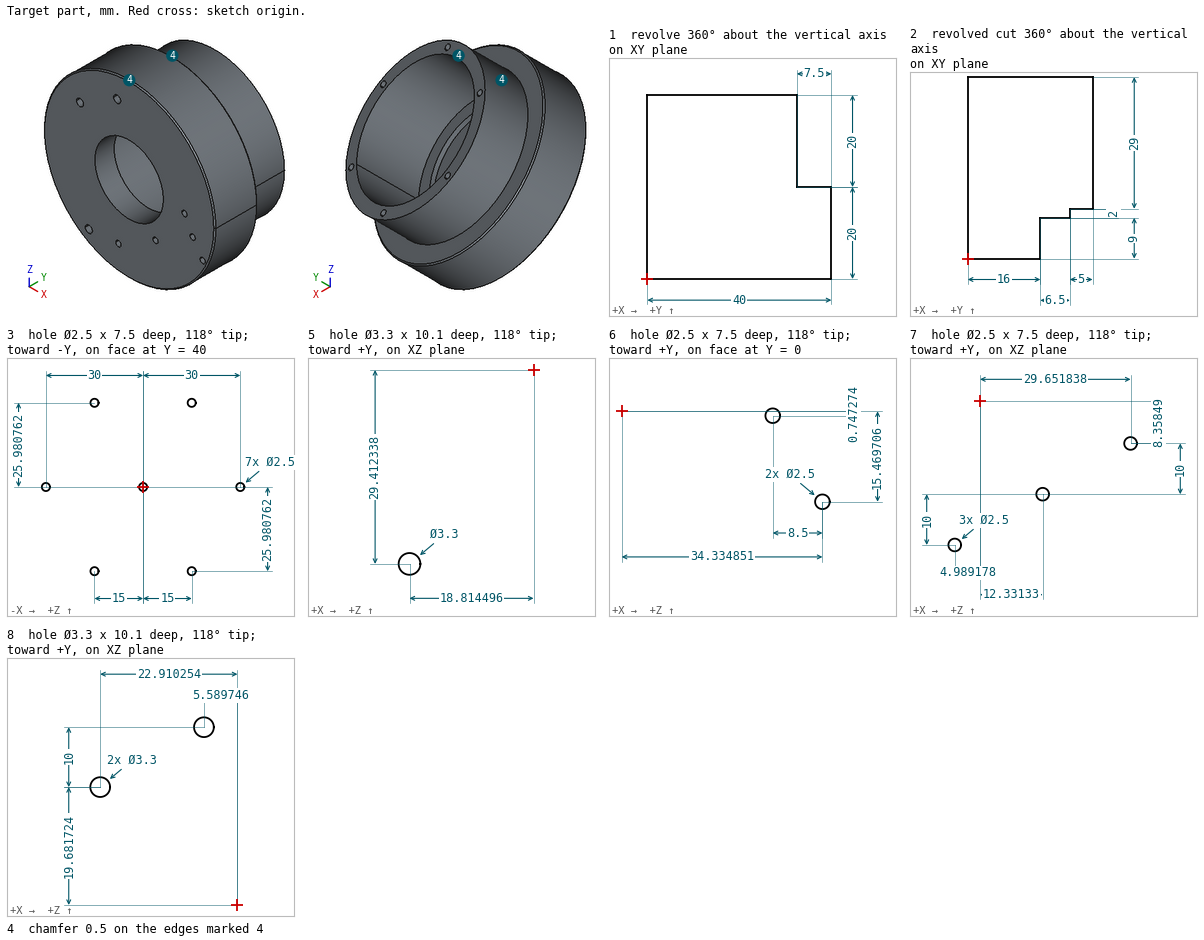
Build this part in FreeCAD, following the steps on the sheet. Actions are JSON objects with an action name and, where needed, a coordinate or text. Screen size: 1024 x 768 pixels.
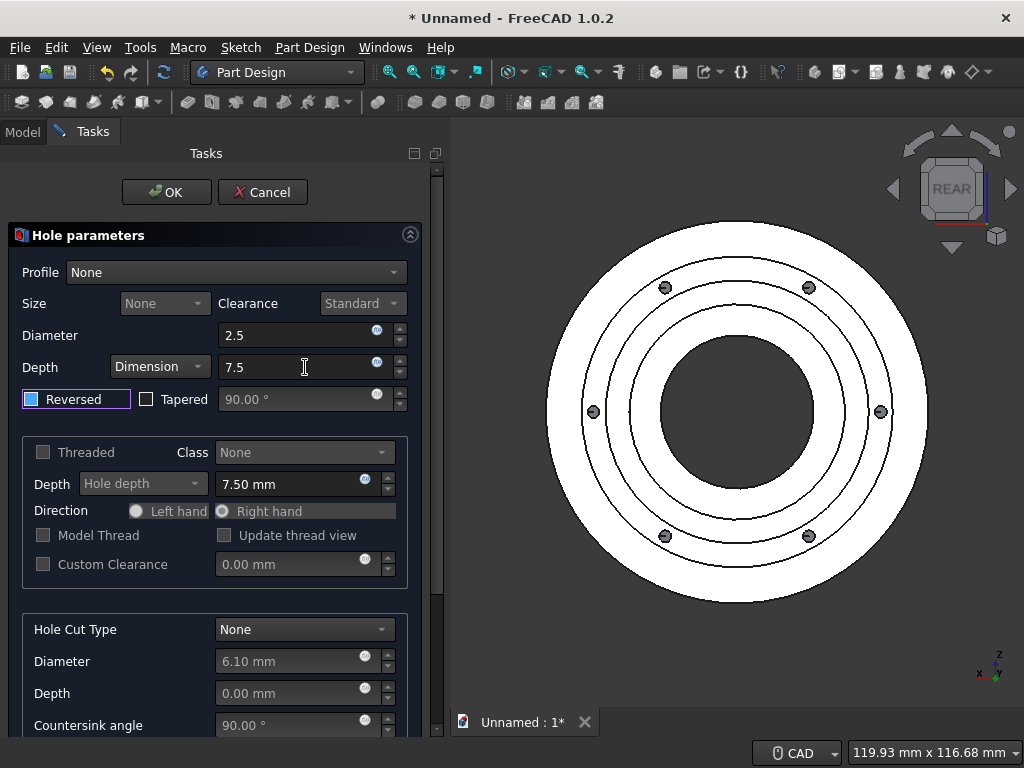
{"action": "left_click", "coordinate": [167, 192]}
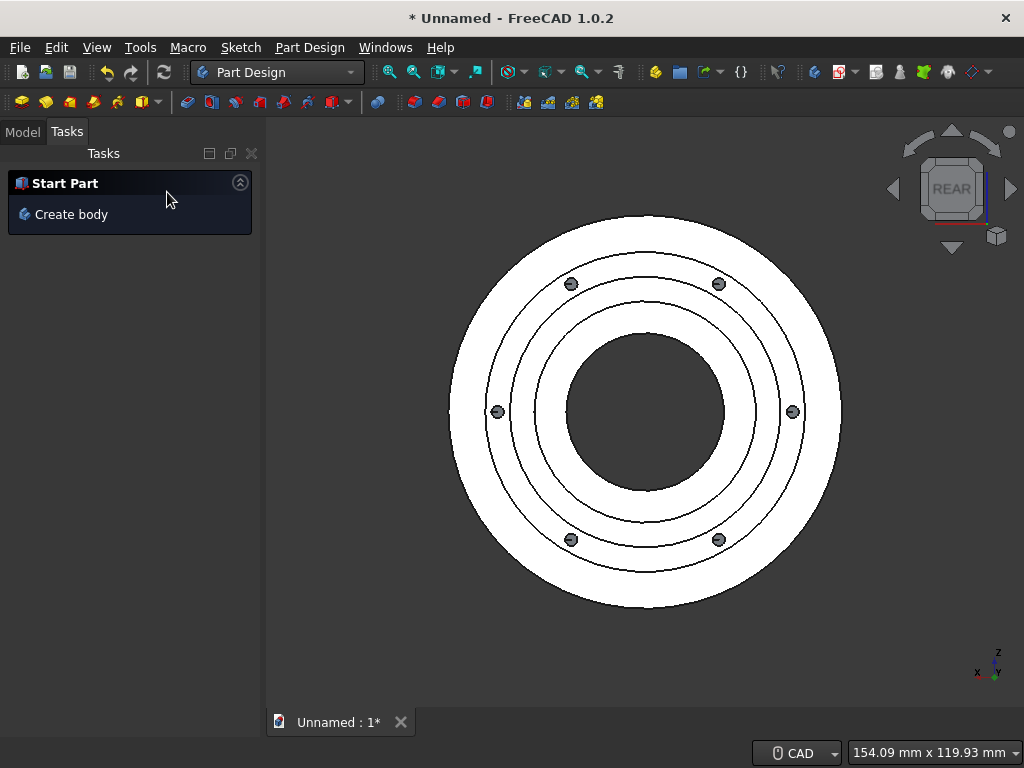
{"action": "left_click", "coordinate": [842, 411]}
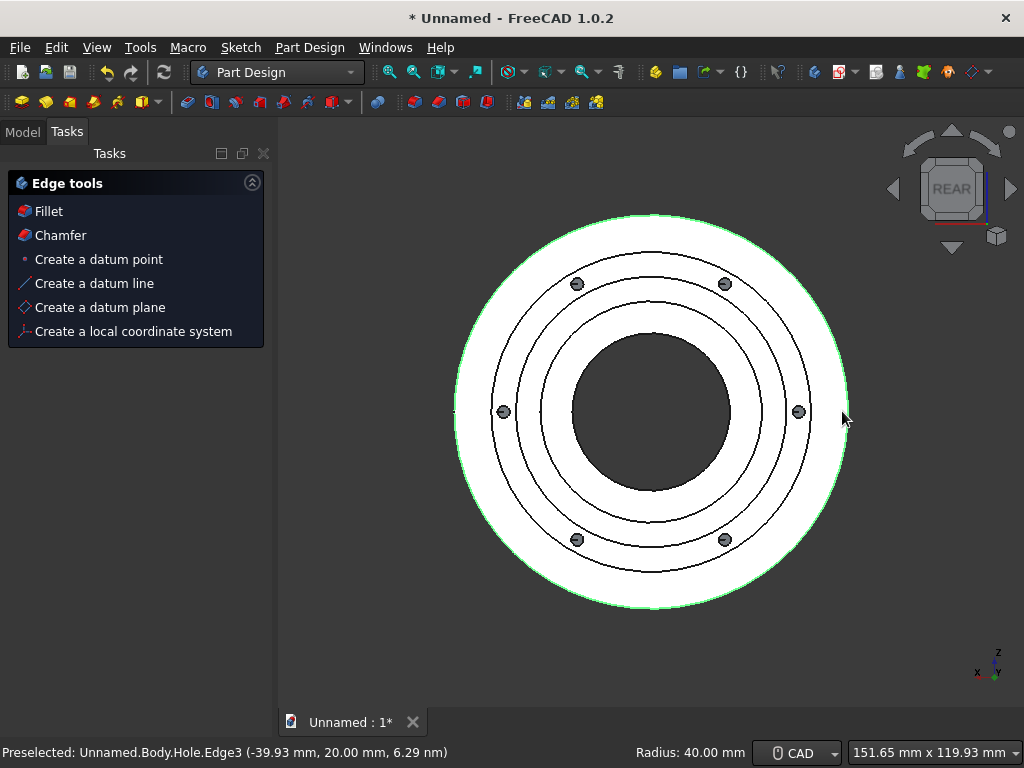
{"action": "key", "text": "0"}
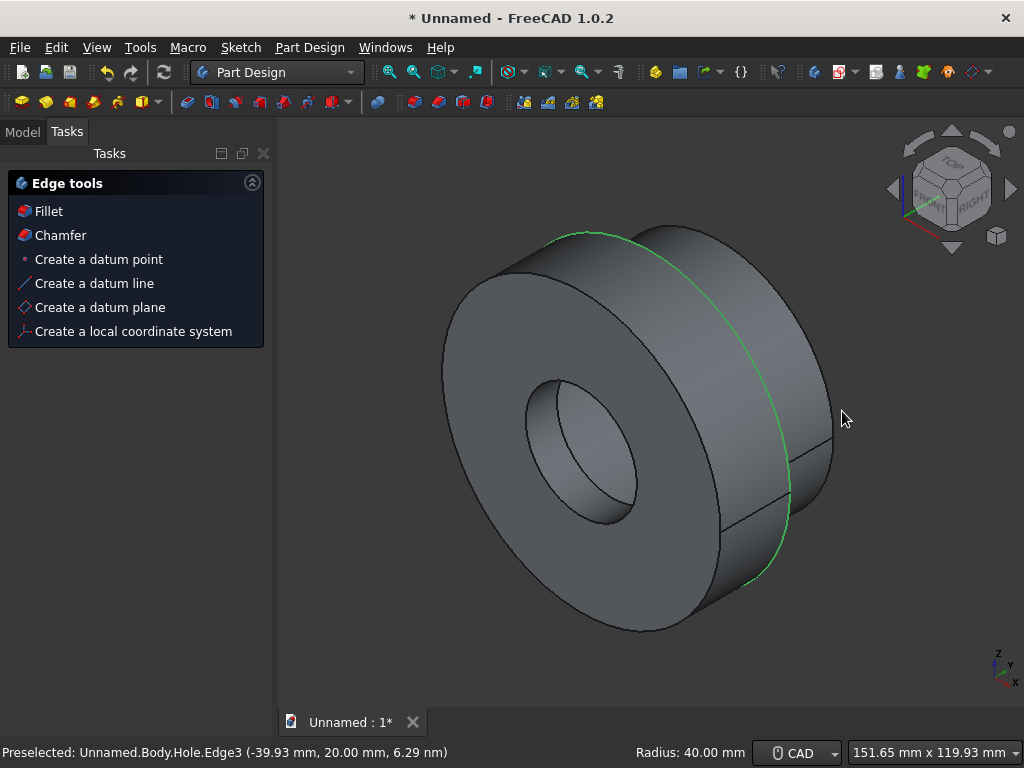
{"action": "left_click", "coordinate": [538, 273], "text": "ctrl"}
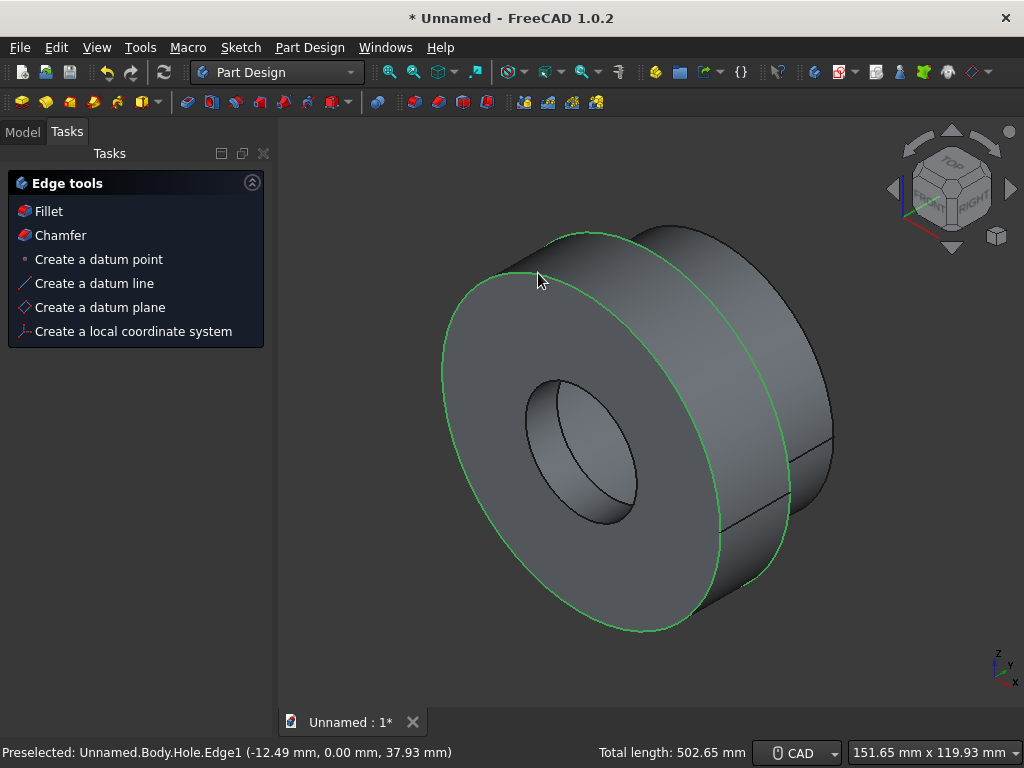
{"action": "left_click", "coordinate": [440, 102]}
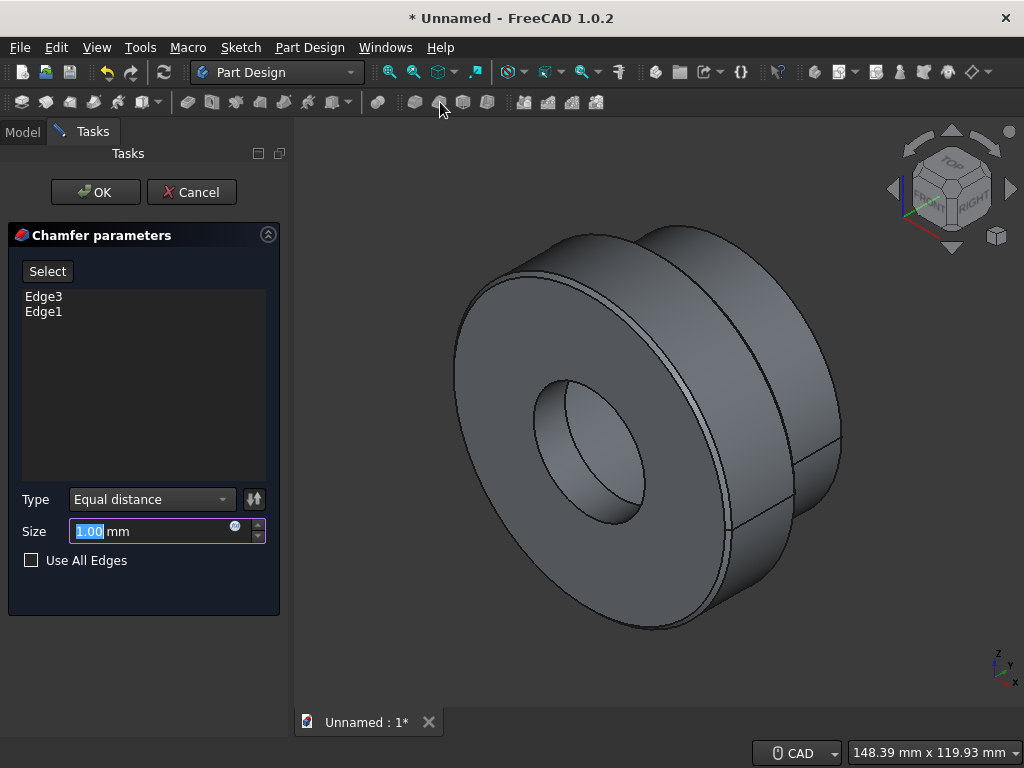
{"action": "type", "text": "0.5"}
{"action": "key", "text": "Tab"}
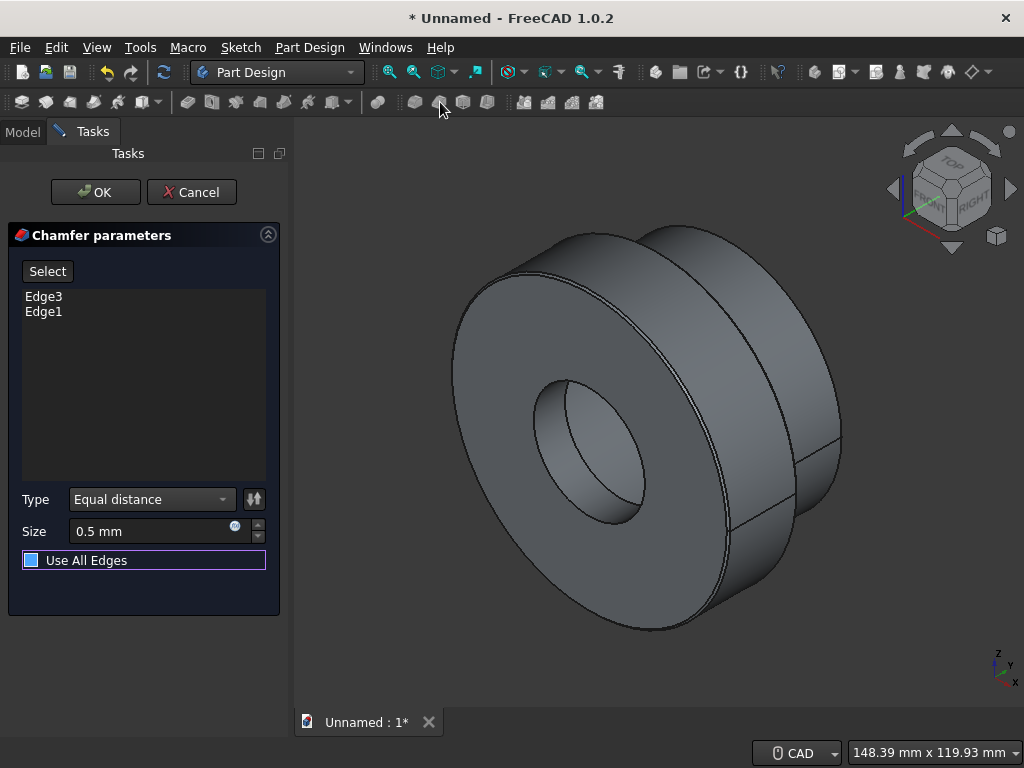
{"action": "left_click", "coordinate": [96, 192]}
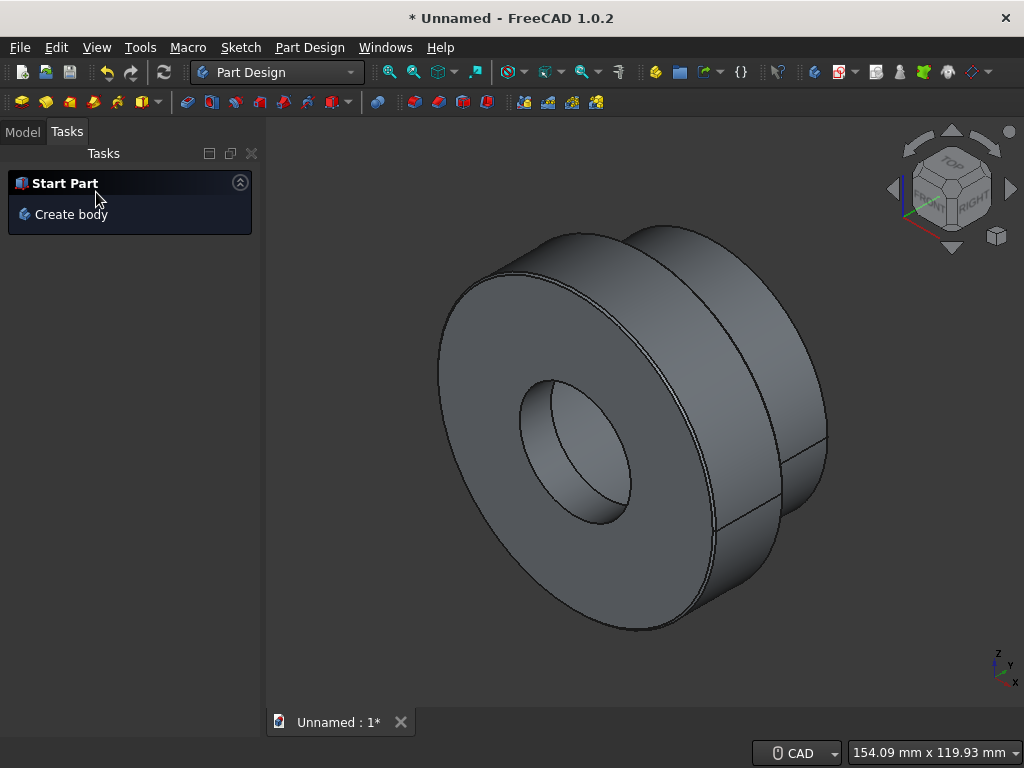
{"action": "left_click", "coordinate": [840, 72]}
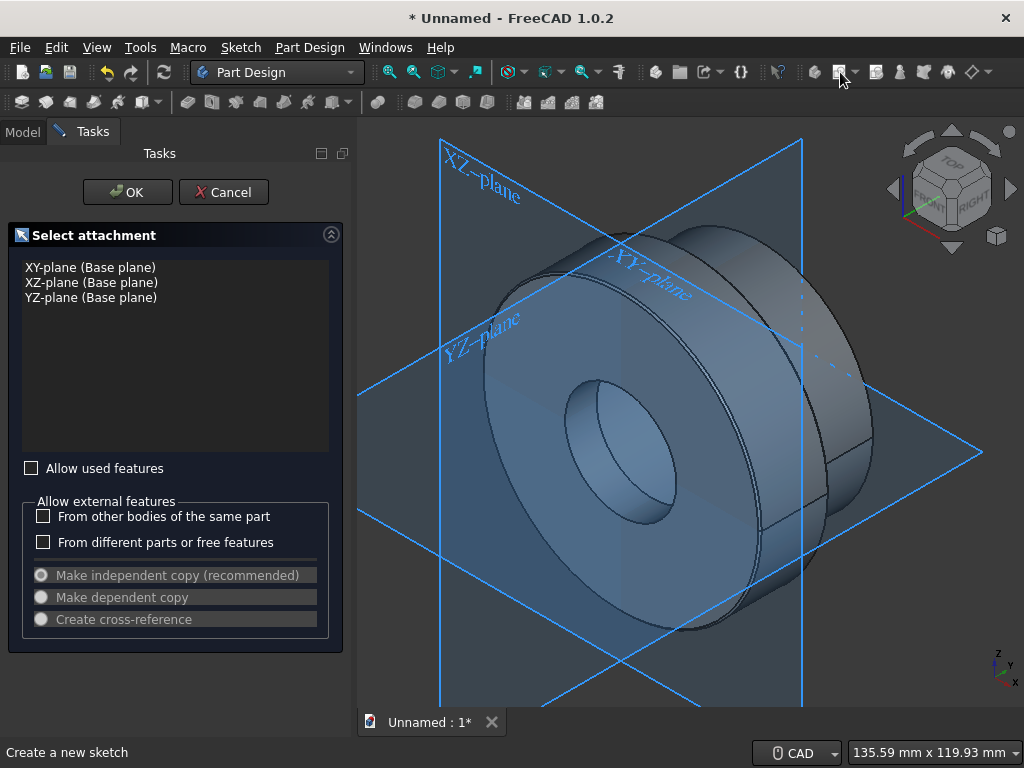
{"action": "left_click", "coordinate": [82, 282]}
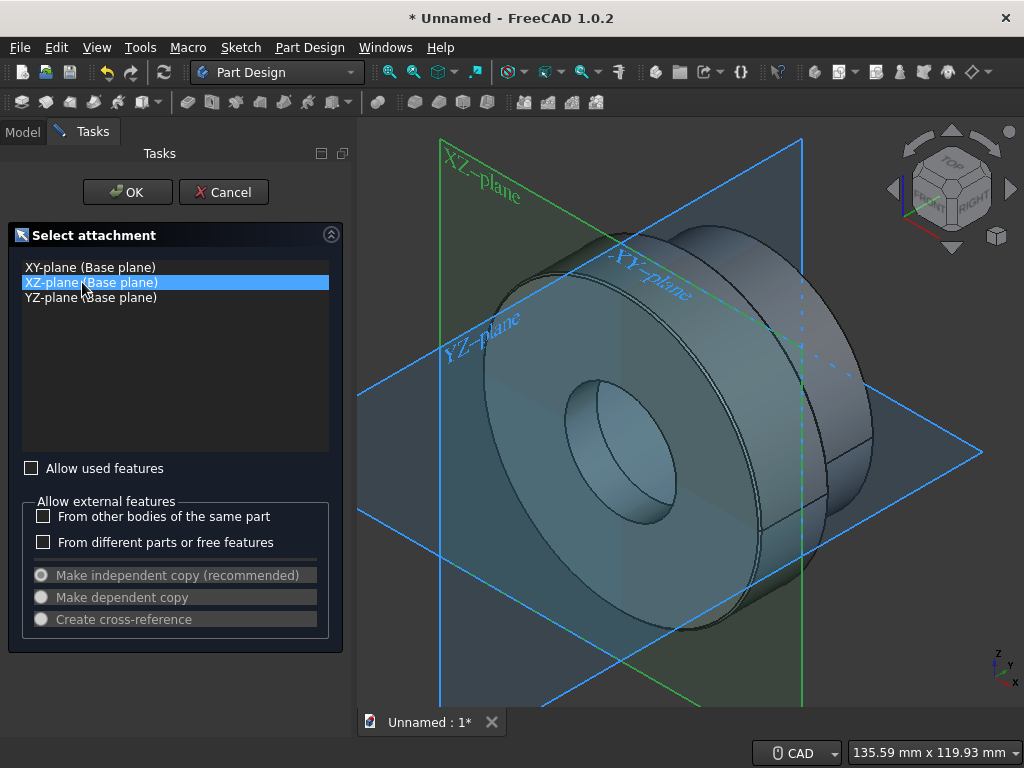
{"action": "left_click", "coordinate": [128, 192]}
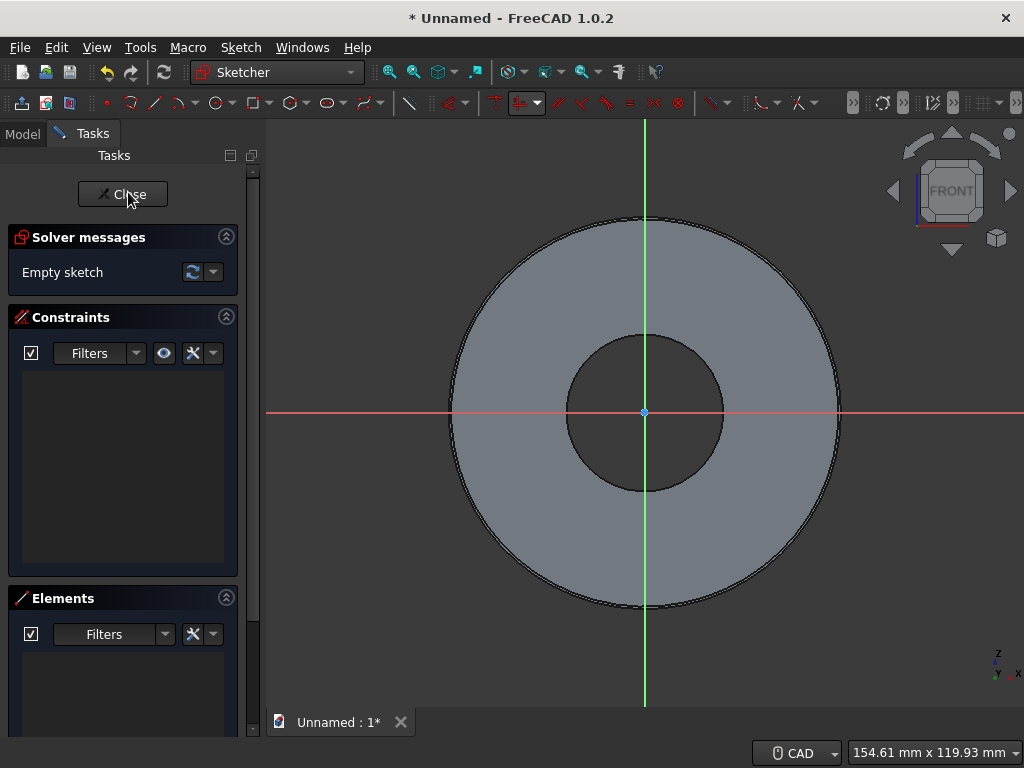
{"action": "scroll", "coordinate": [551, 565], "scroll_direction": "up", "scroll_amount": 15}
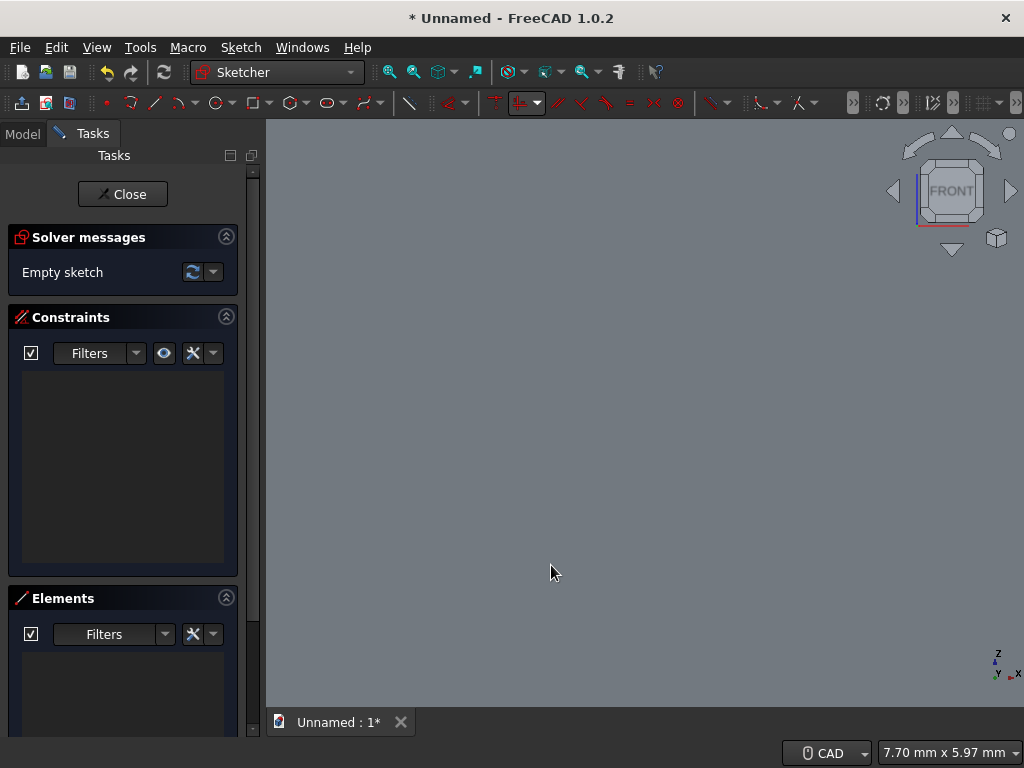
{"action": "left_click", "coordinate": [216, 104]}